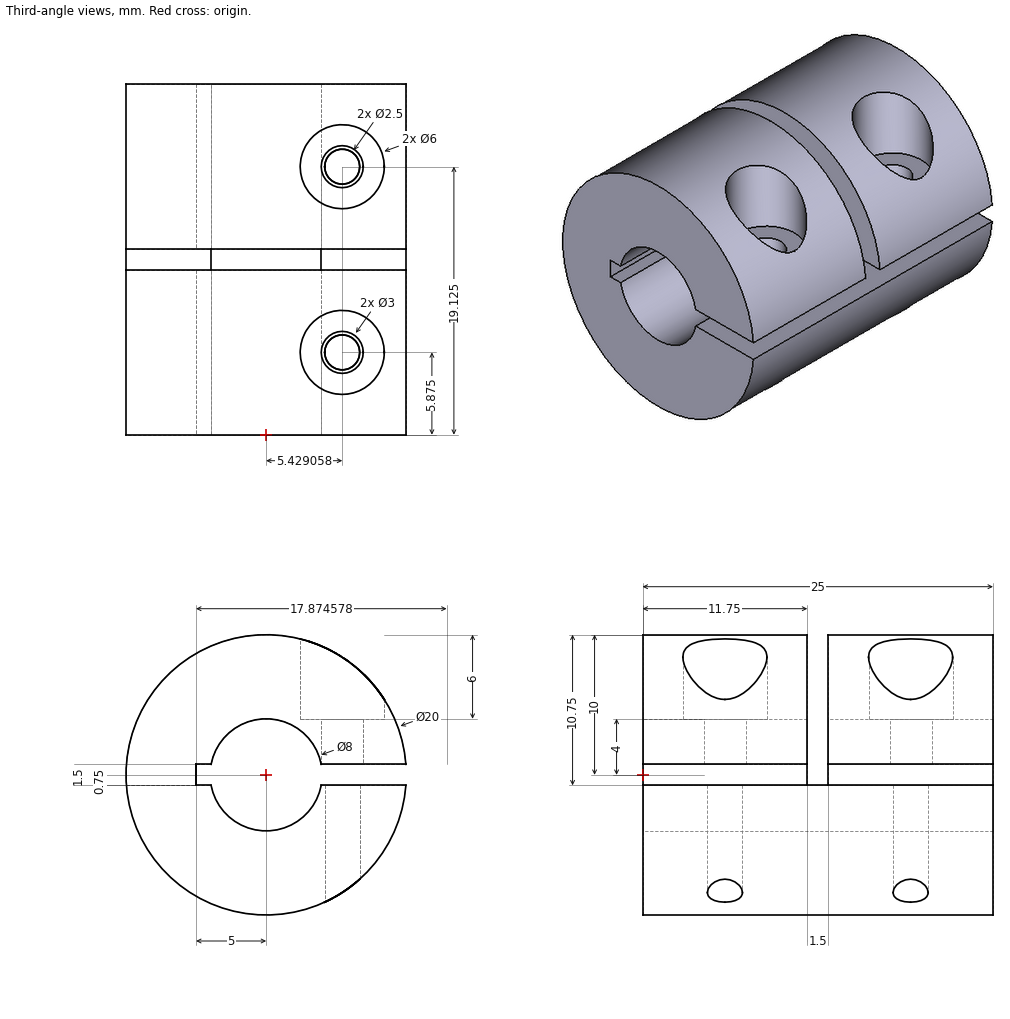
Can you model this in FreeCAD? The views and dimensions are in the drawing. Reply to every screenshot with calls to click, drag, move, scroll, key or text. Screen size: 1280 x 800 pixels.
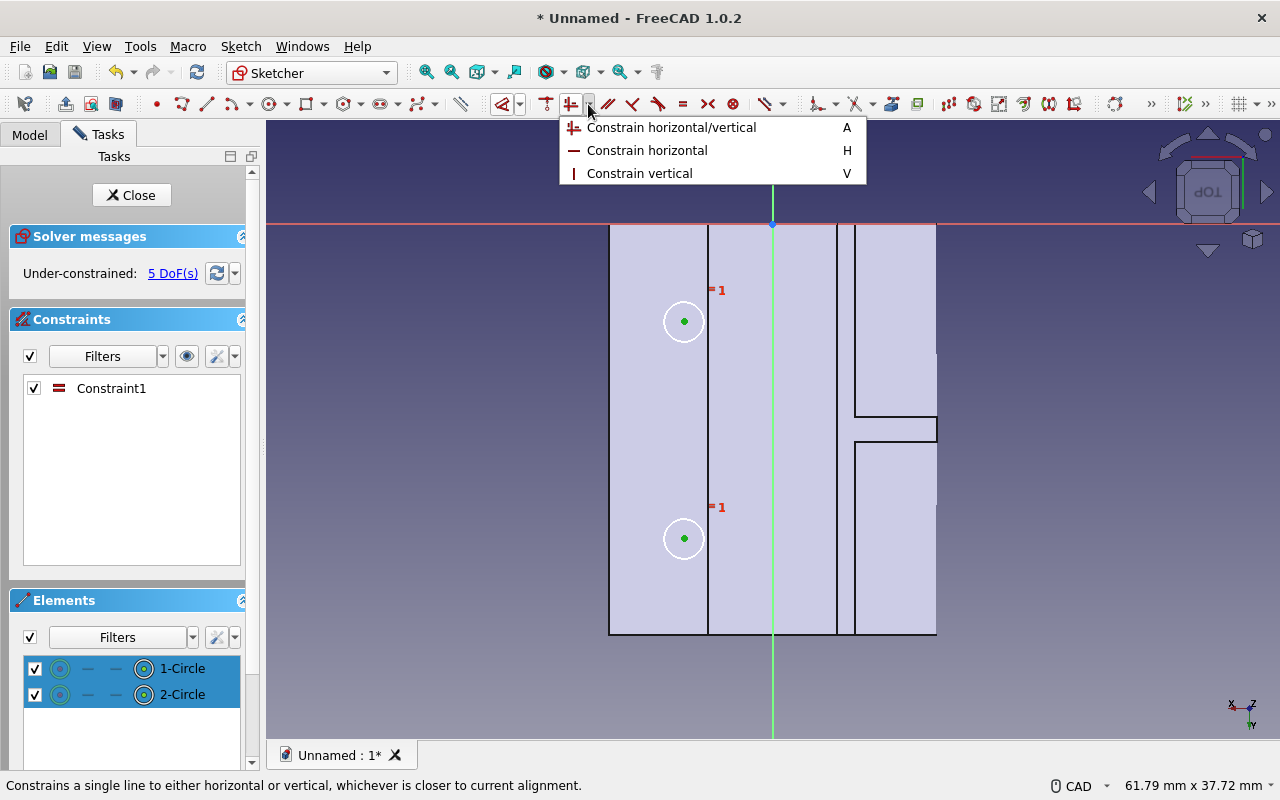
click(713, 174)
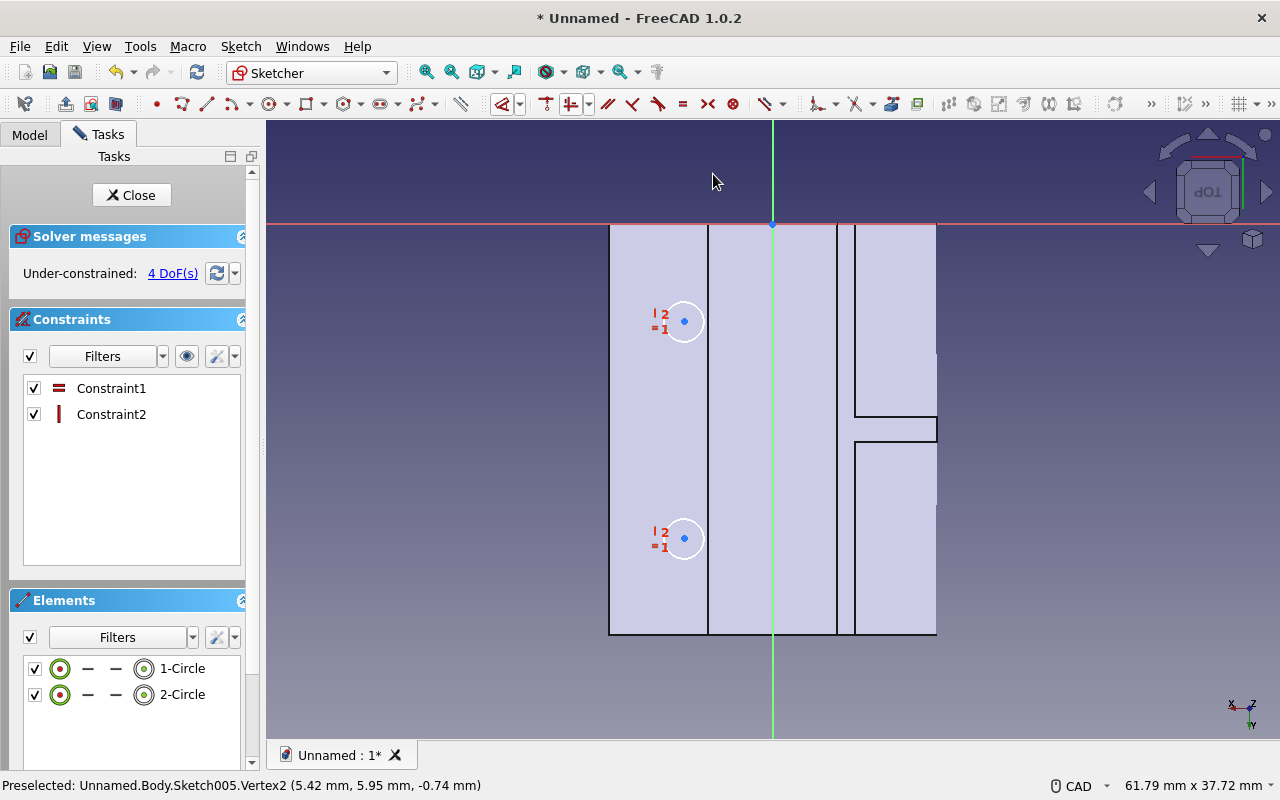
click(698, 525)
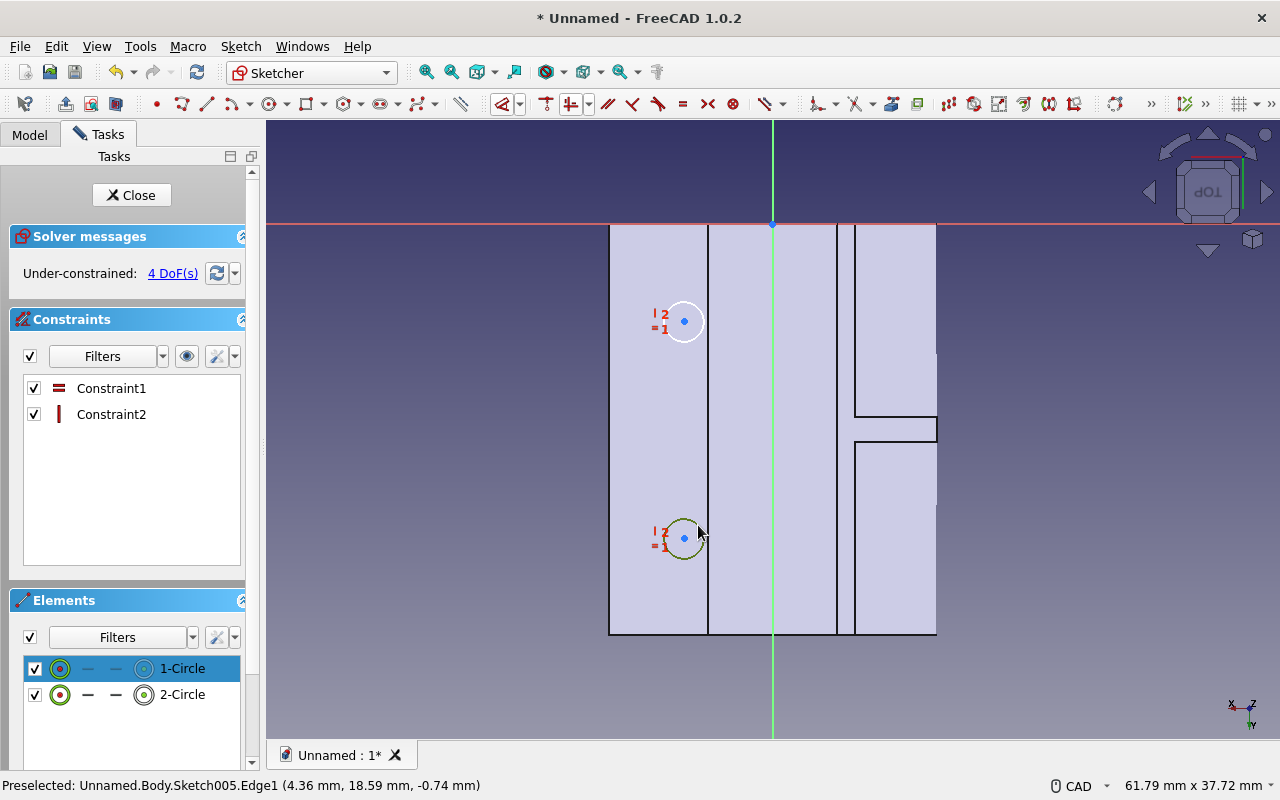
click(520, 104)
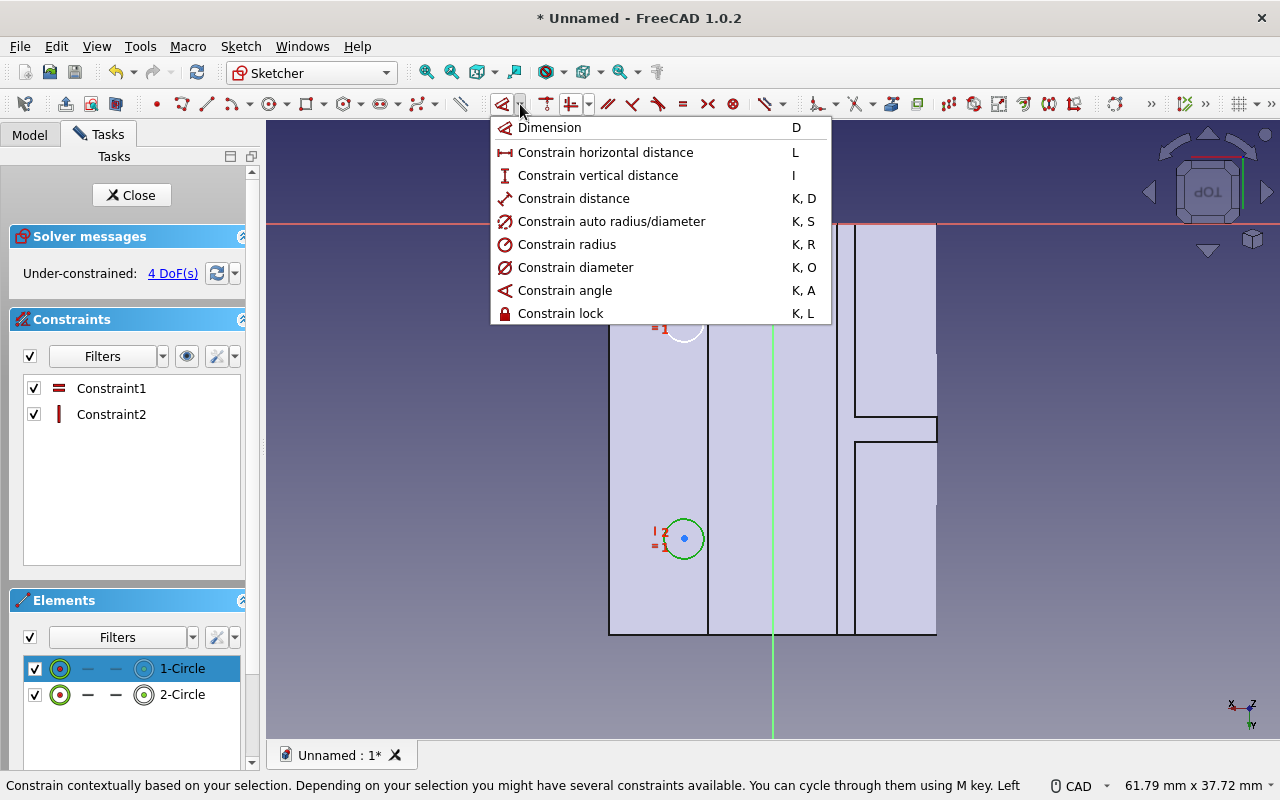
click(661, 268)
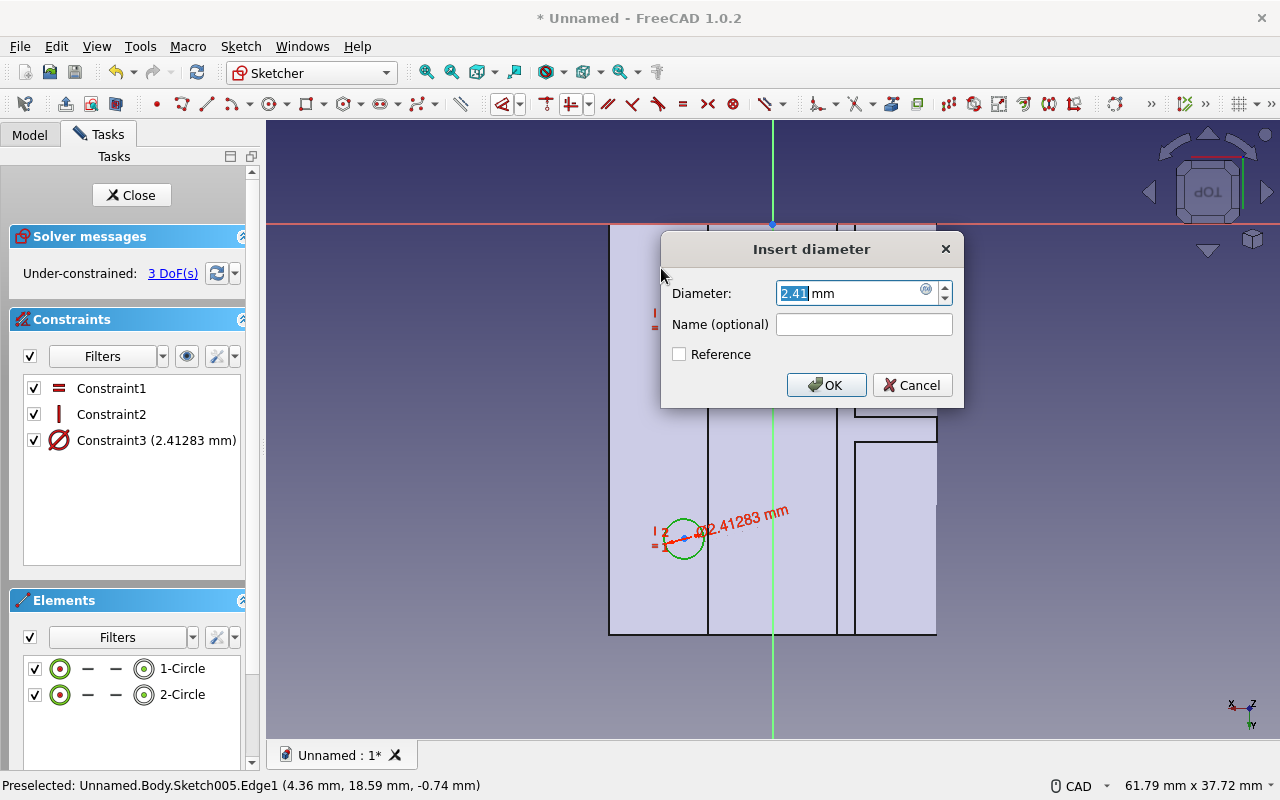
text(2.5)
key(Return)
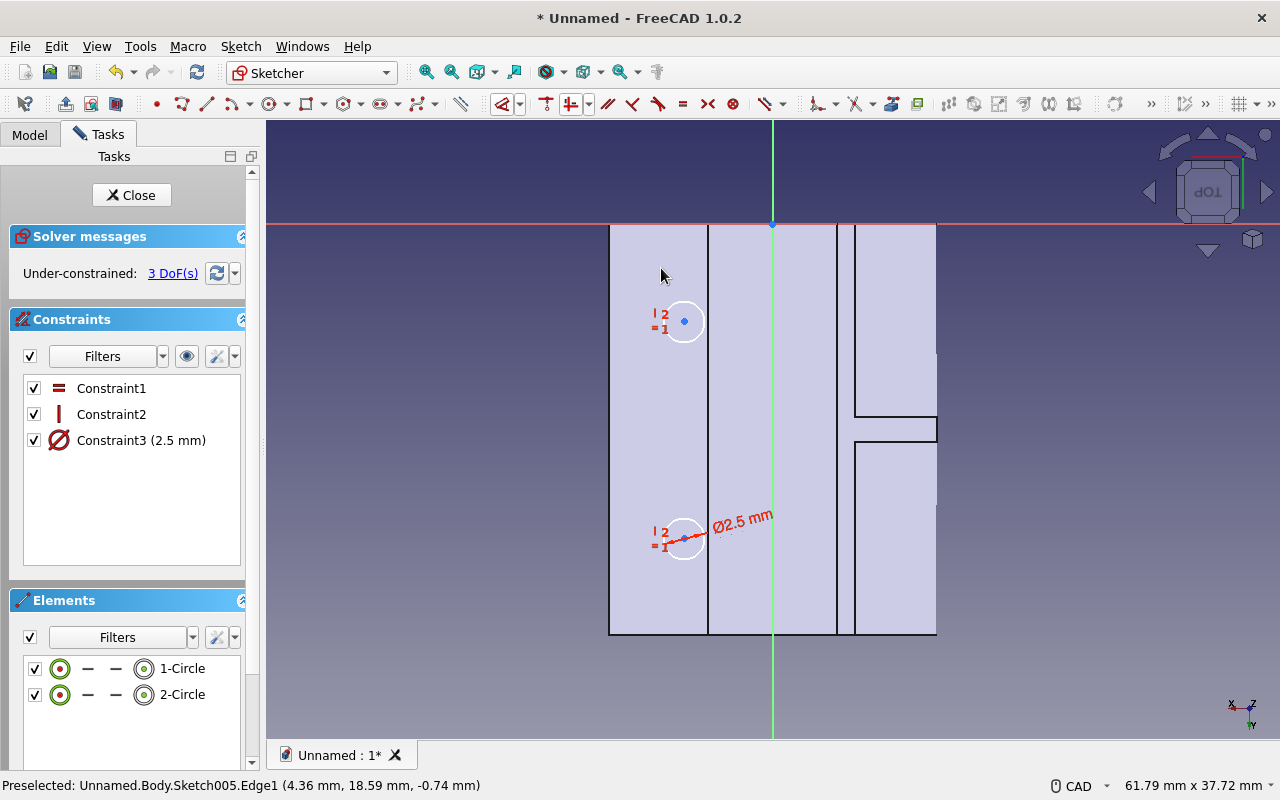
click(684, 322)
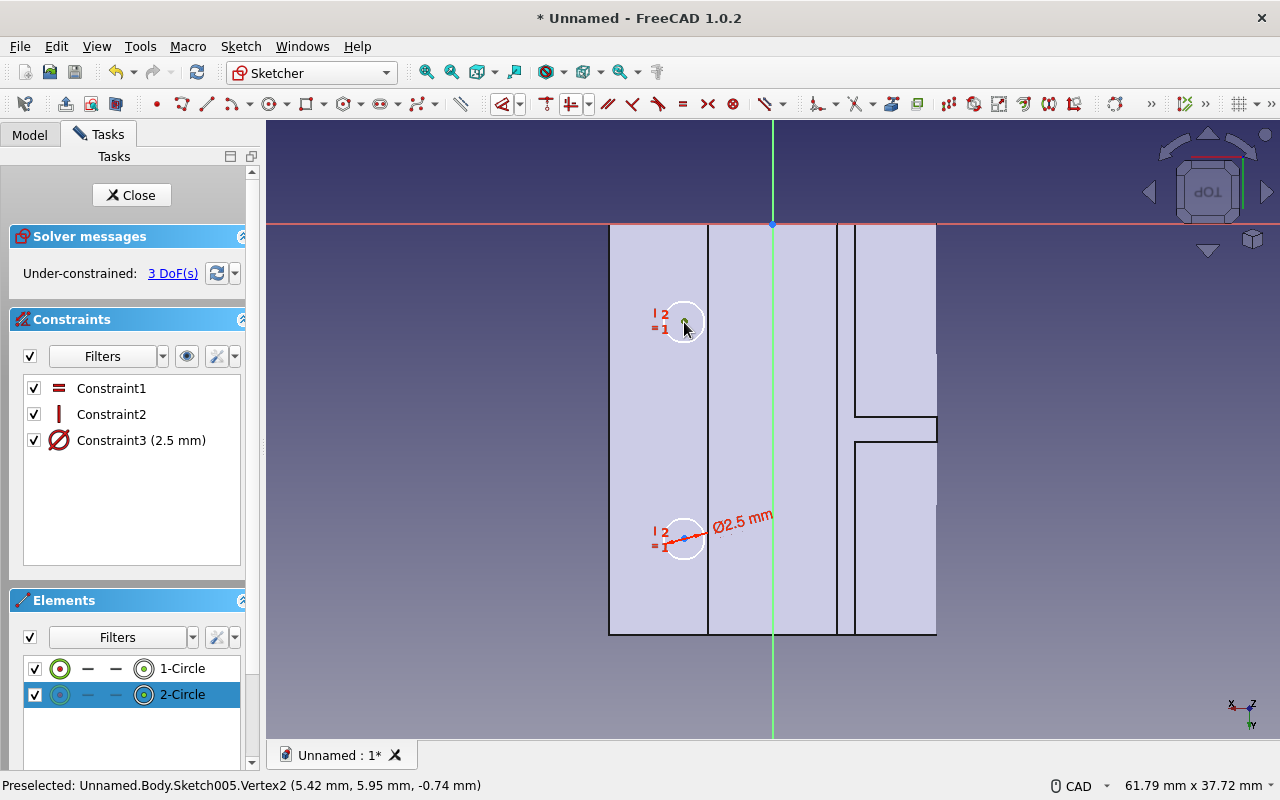
click(520, 104)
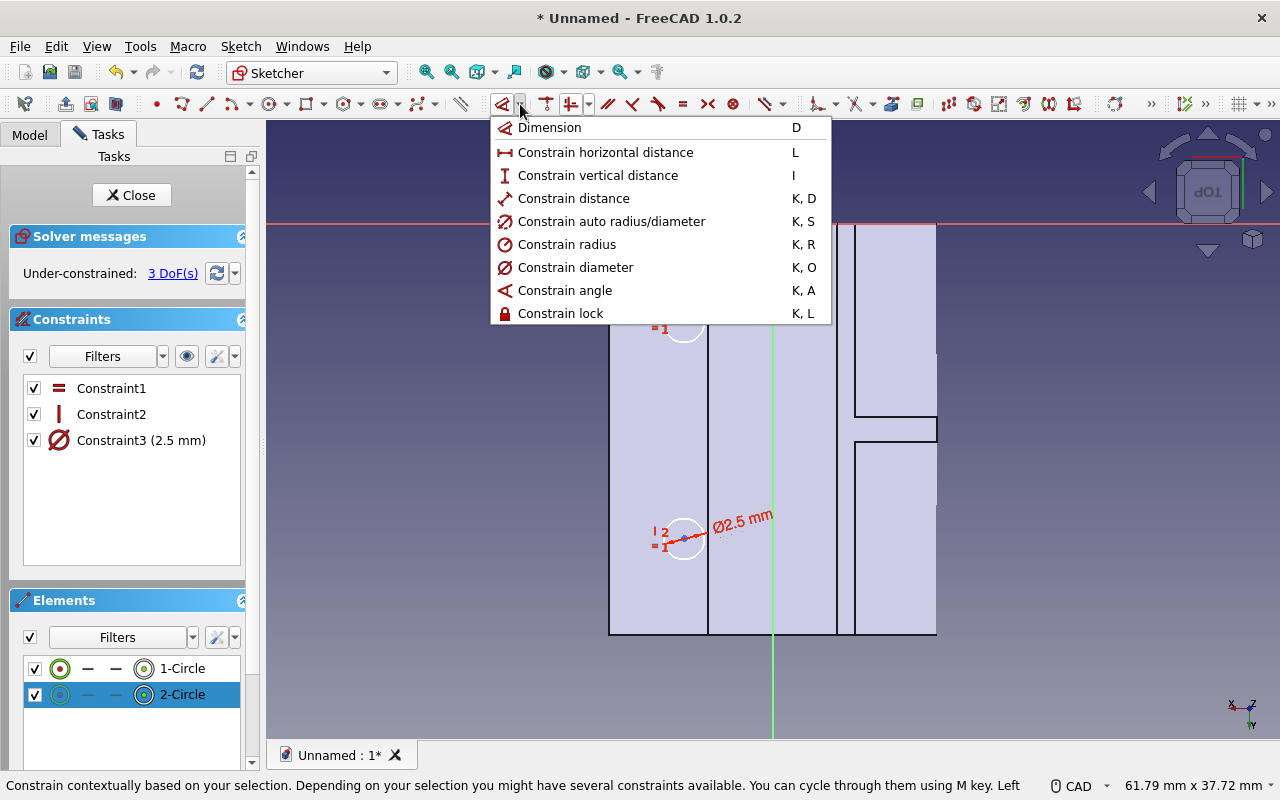
click(661, 176)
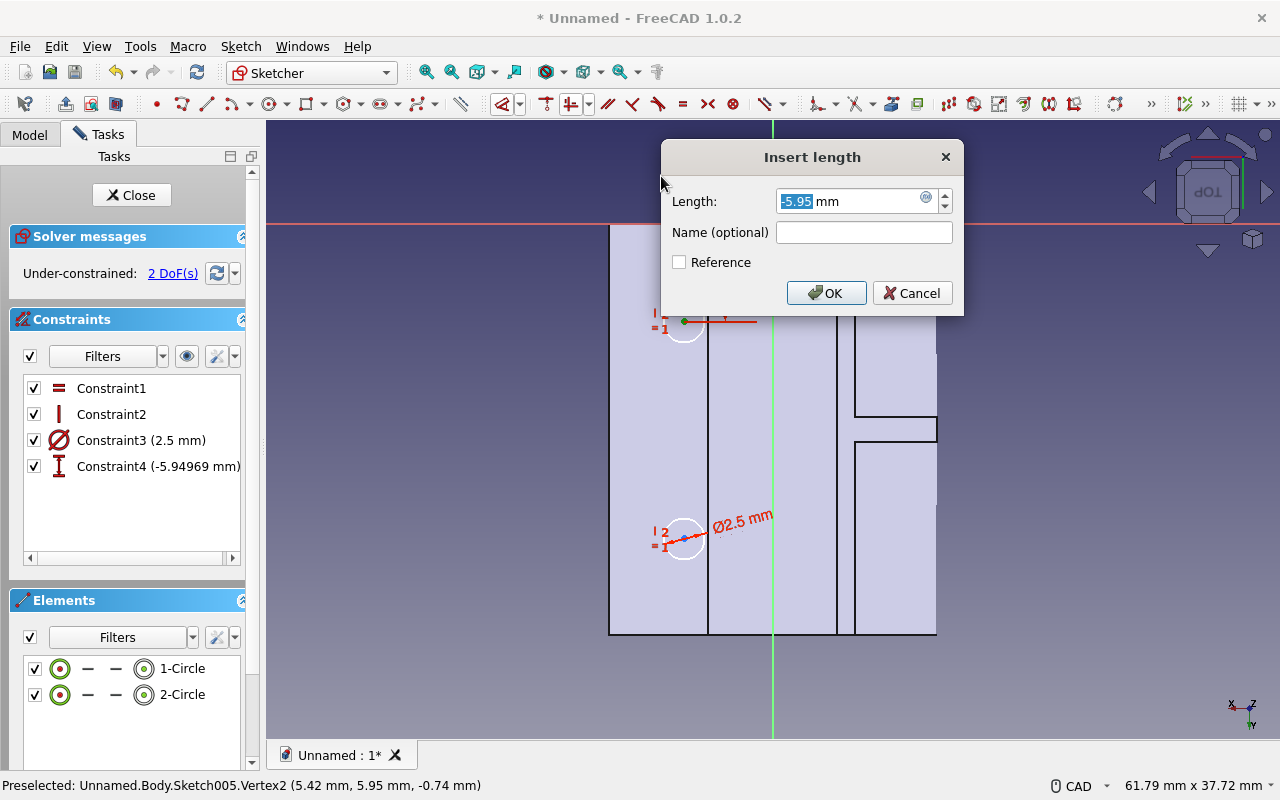
text(-5.875)
key(Return)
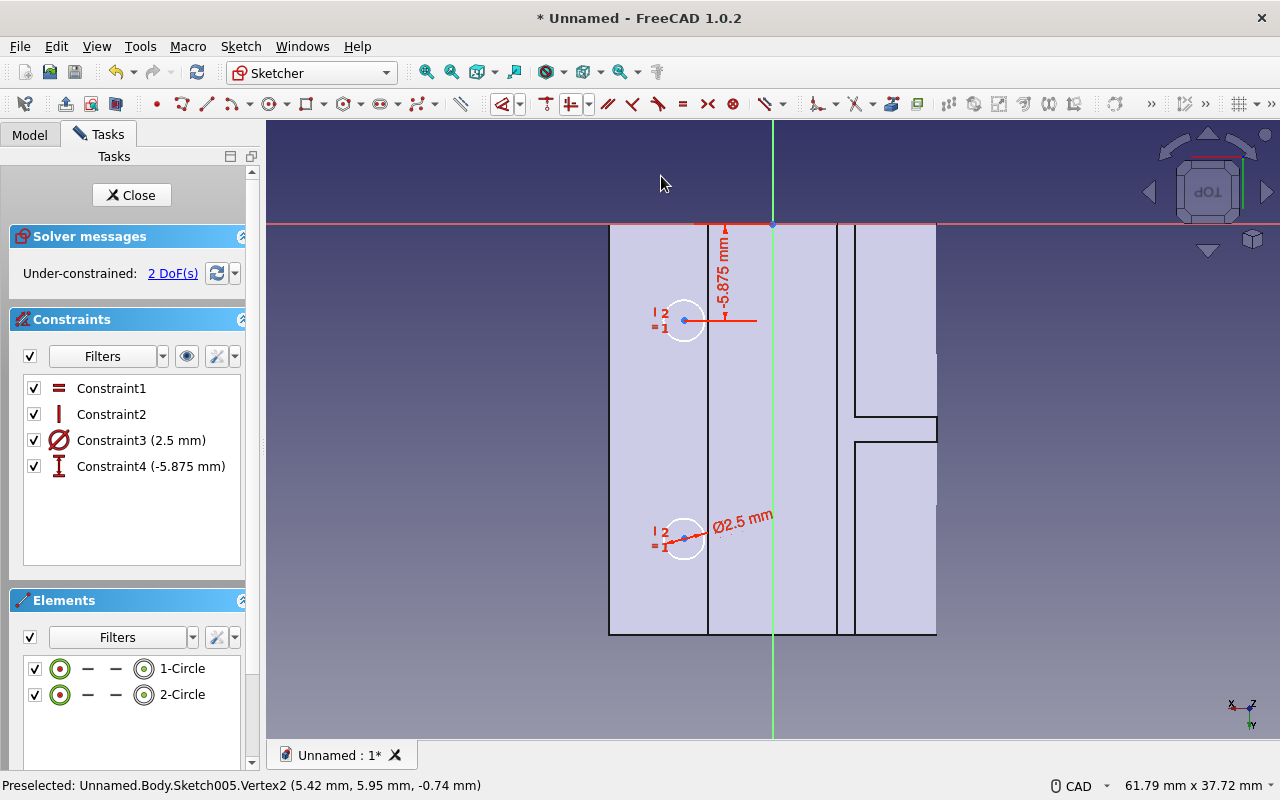
click(684, 539)